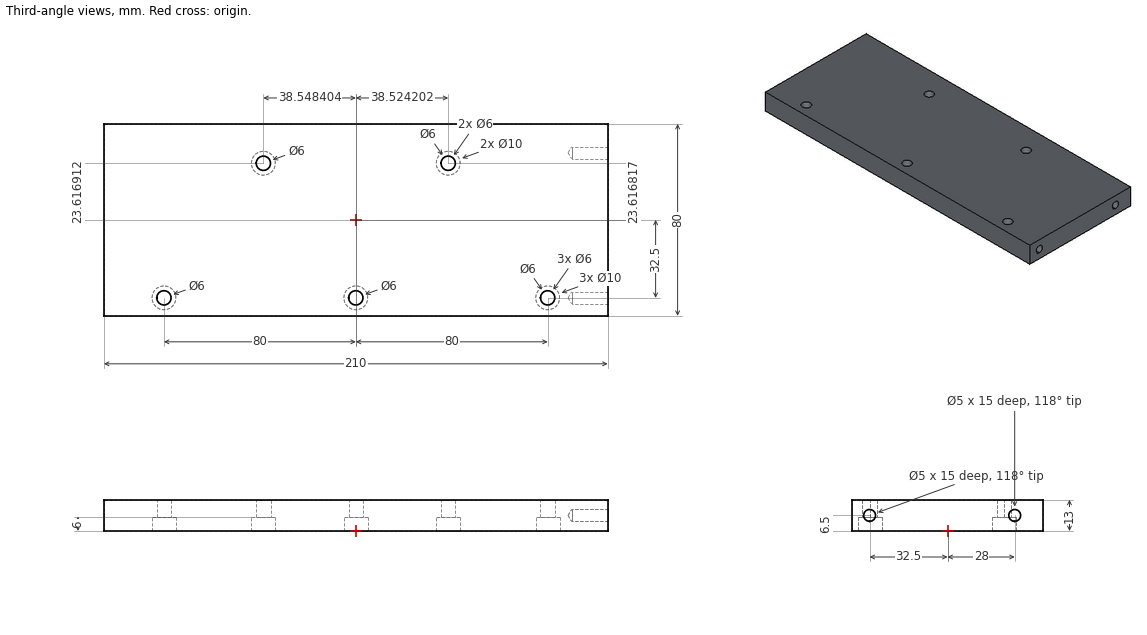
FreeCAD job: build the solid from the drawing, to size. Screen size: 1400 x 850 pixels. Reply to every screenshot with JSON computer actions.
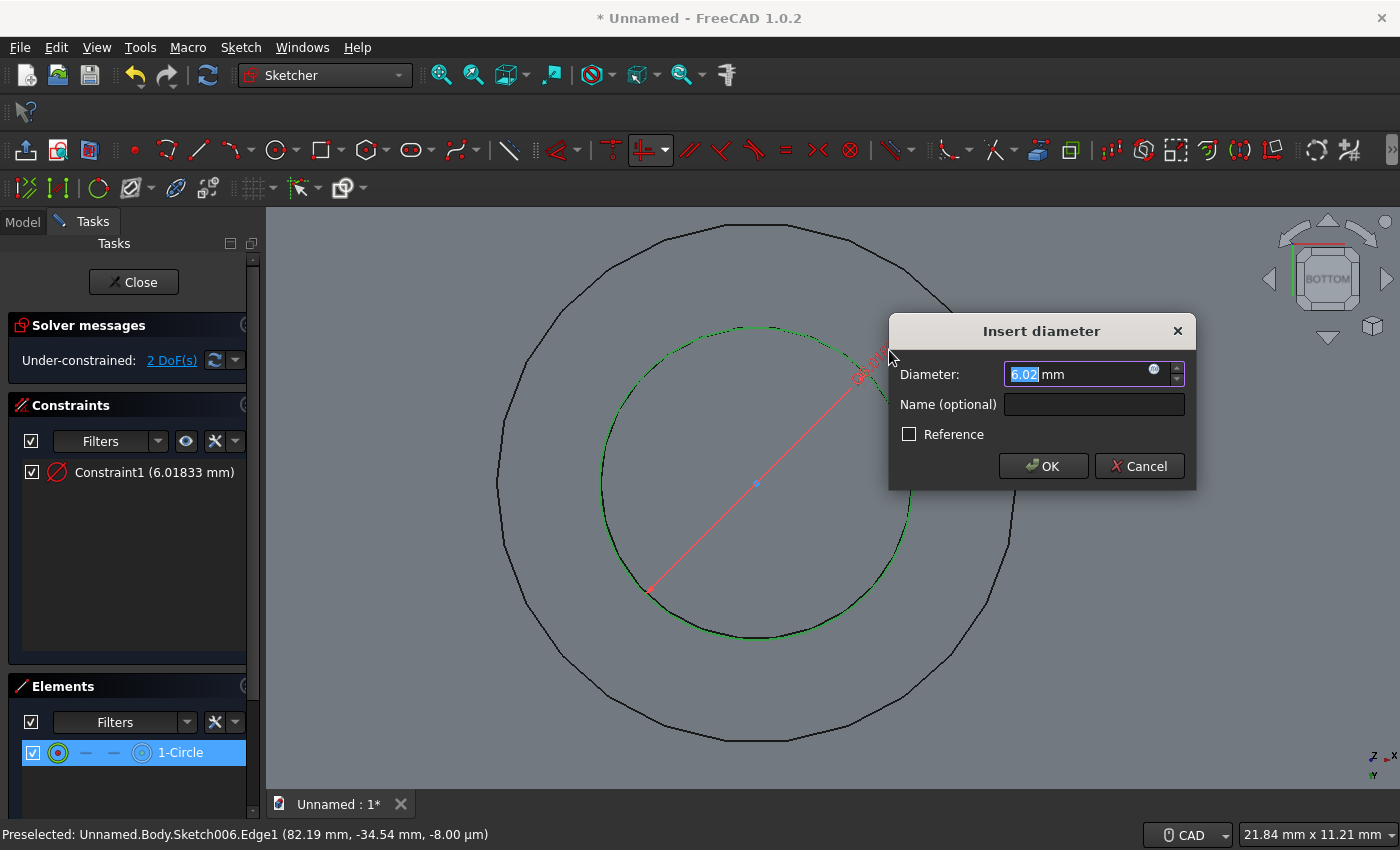
{"action": "type", "text": "6"}
{"action": "key", "text": "Return"}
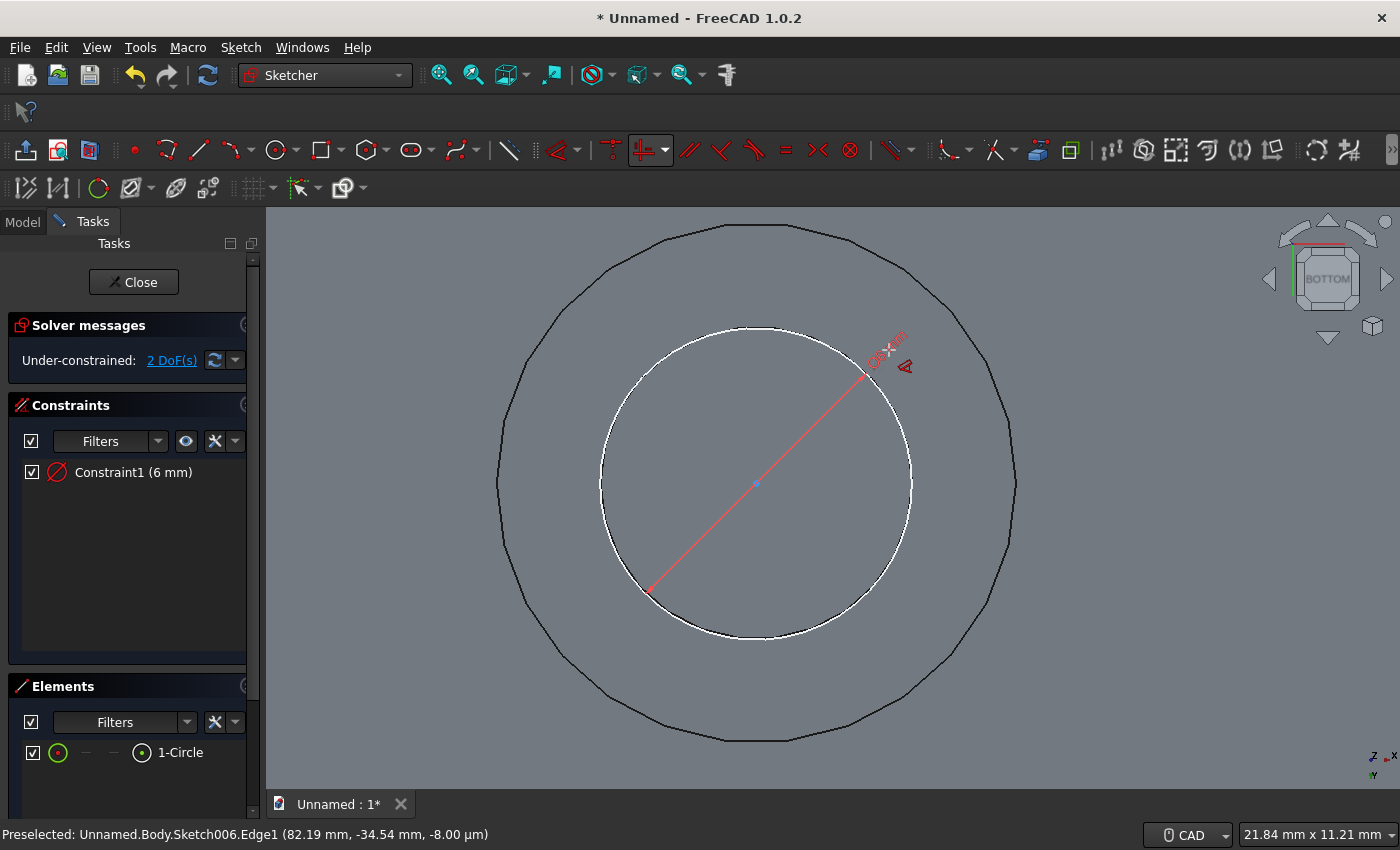
{"action": "left_click", "coordinate": [756, 484]}
{"action": "left_click", "coordinate": [525, 450]}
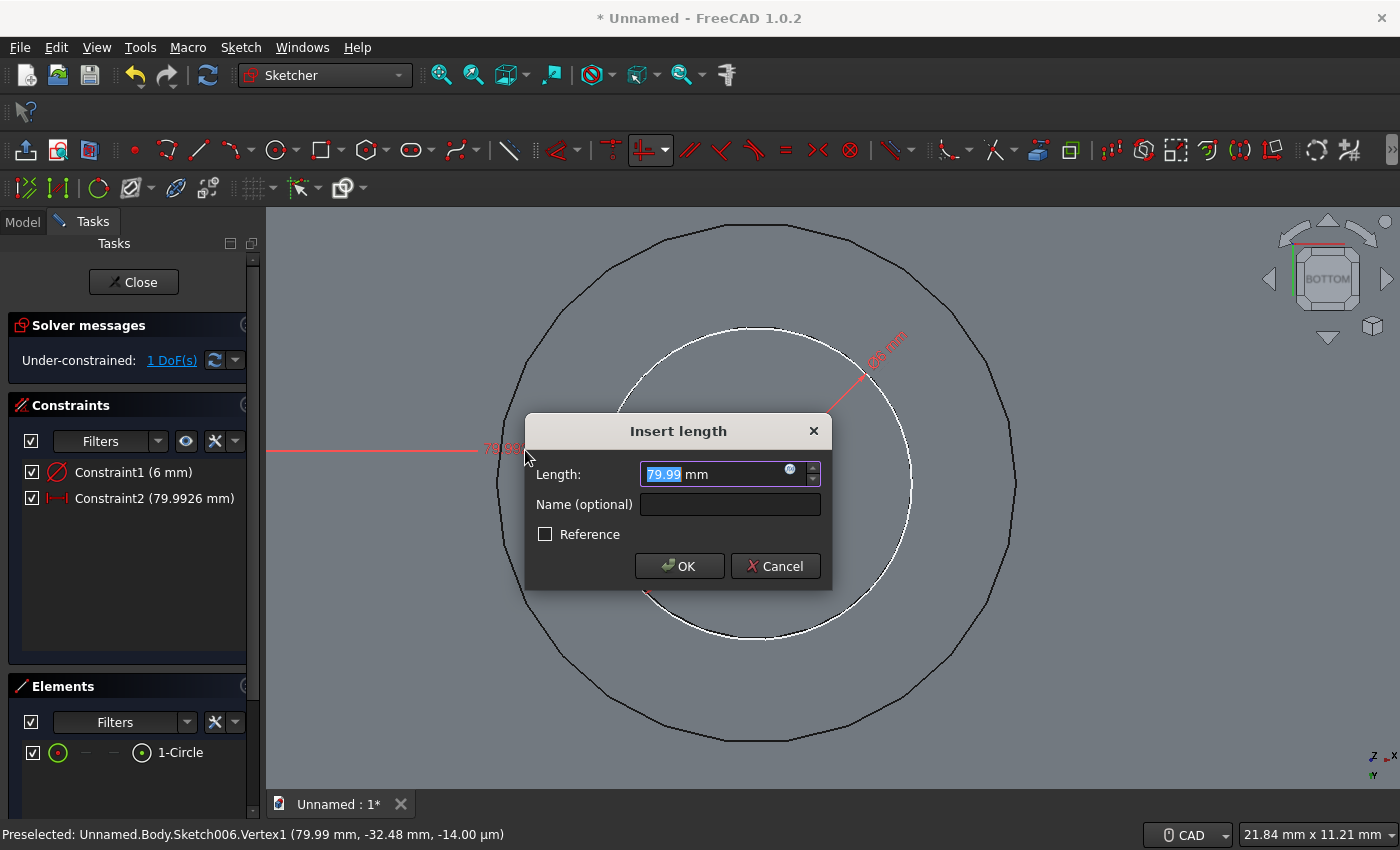
{"action": "type", "text": "80"}
{"action": "key", "text": "Return"}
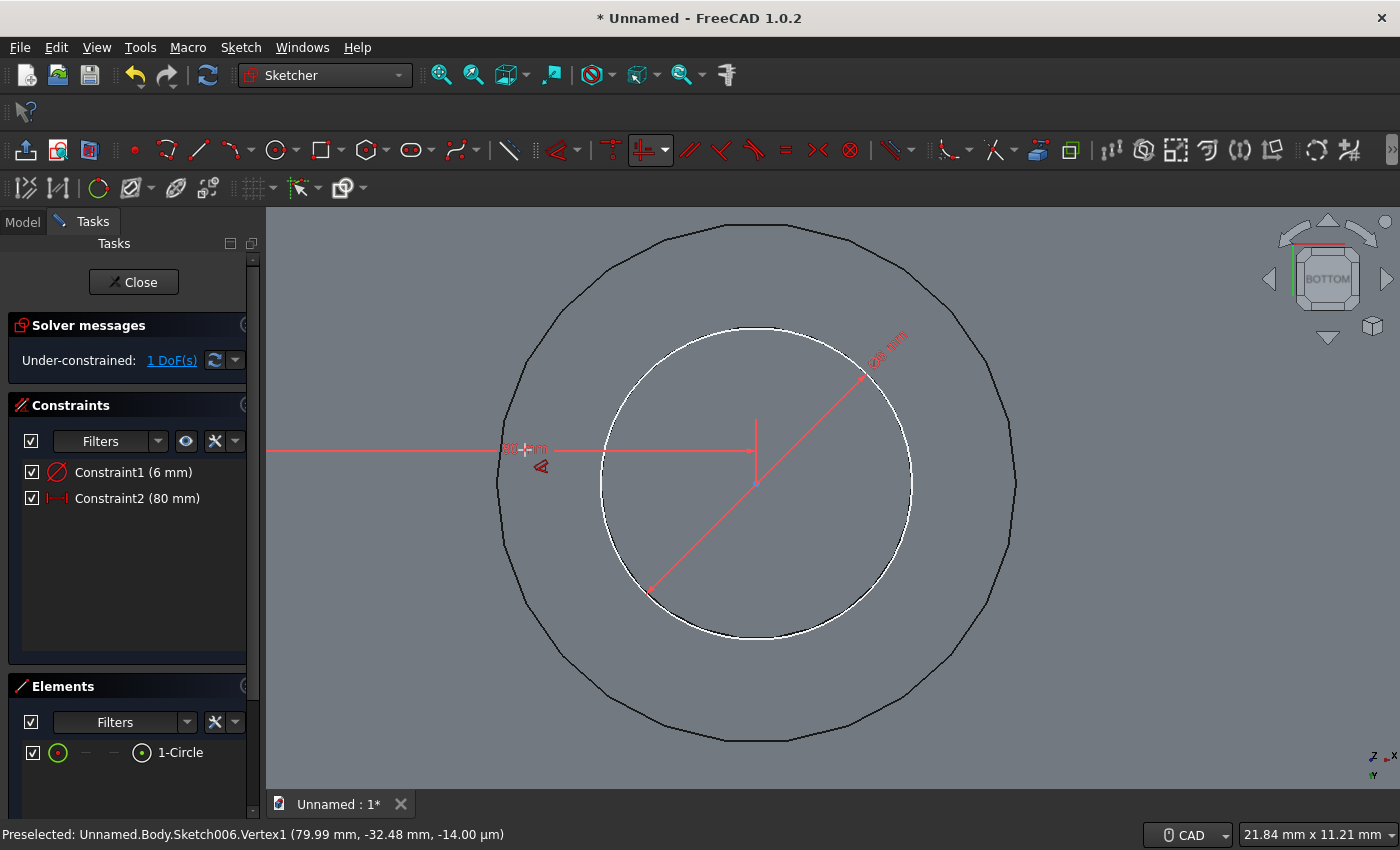
{"action": "left_click", "coordinate": [756, 484]}
{"action": "left_click", "coordinate": [790, 622]}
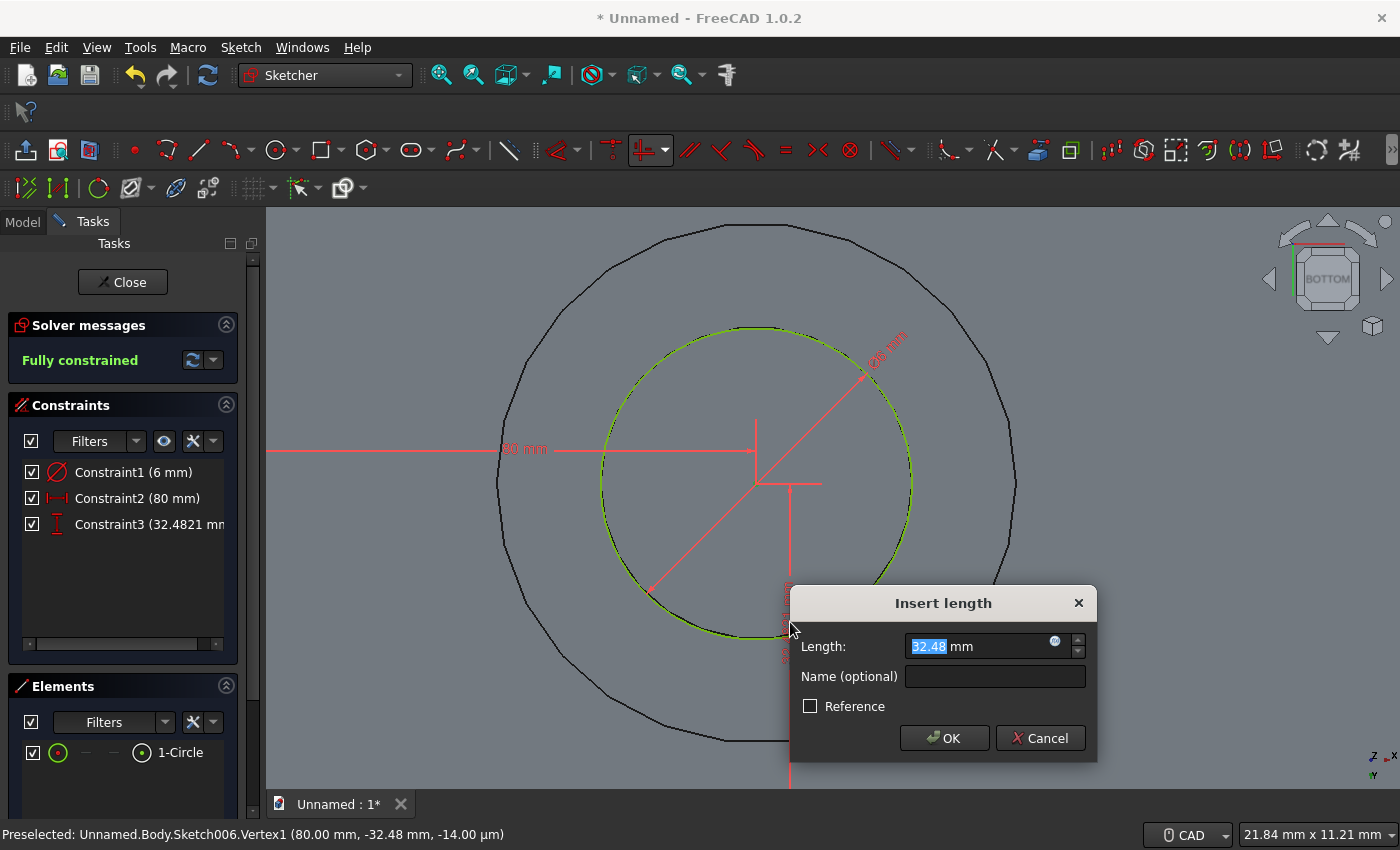
{"action": "type", "text": "32.5"}
{"action": "key", "text": "Return"}
{"action": "key", "text": "Escape"}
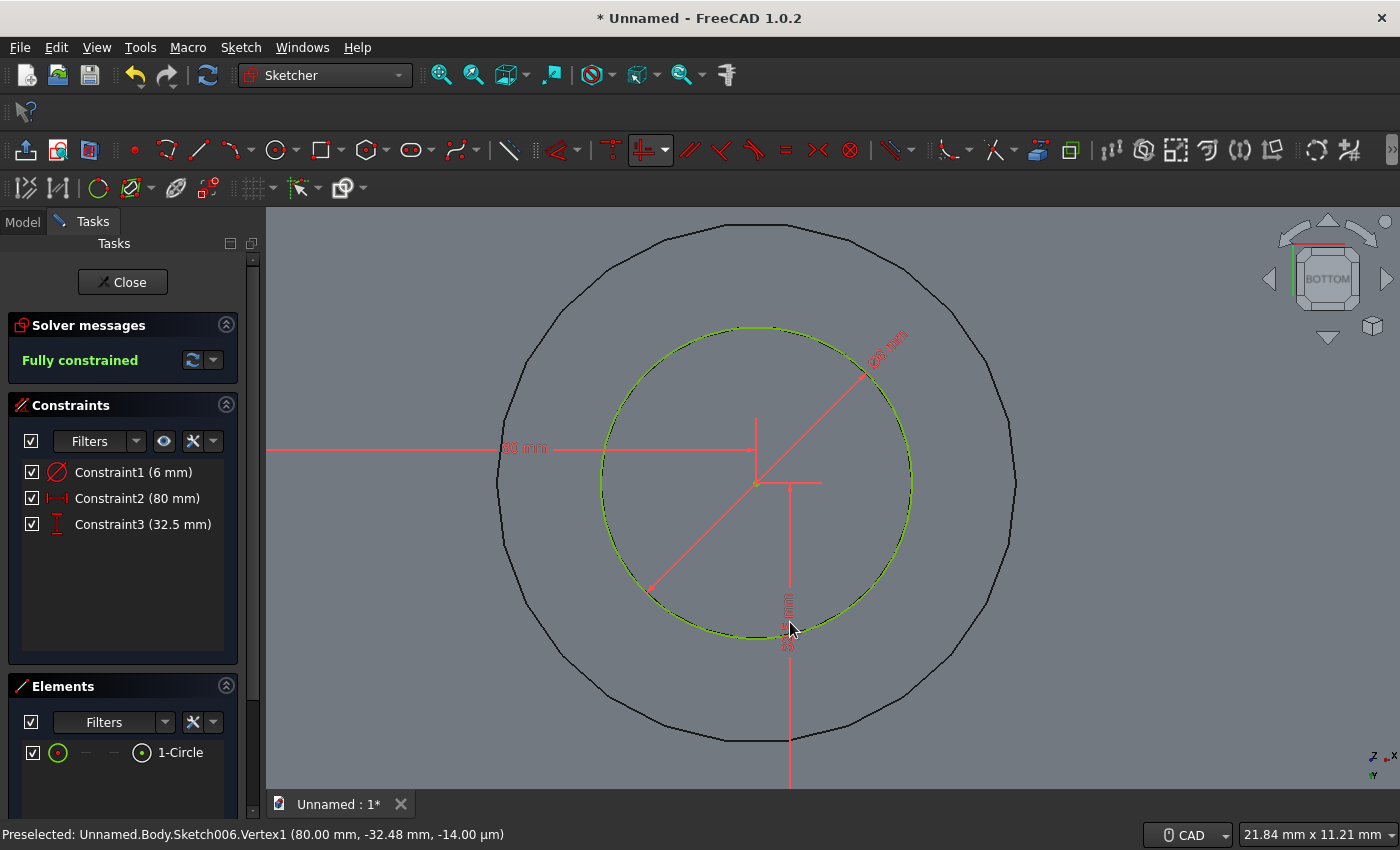
{"action": "left_click", "coordinate": [123, 282]}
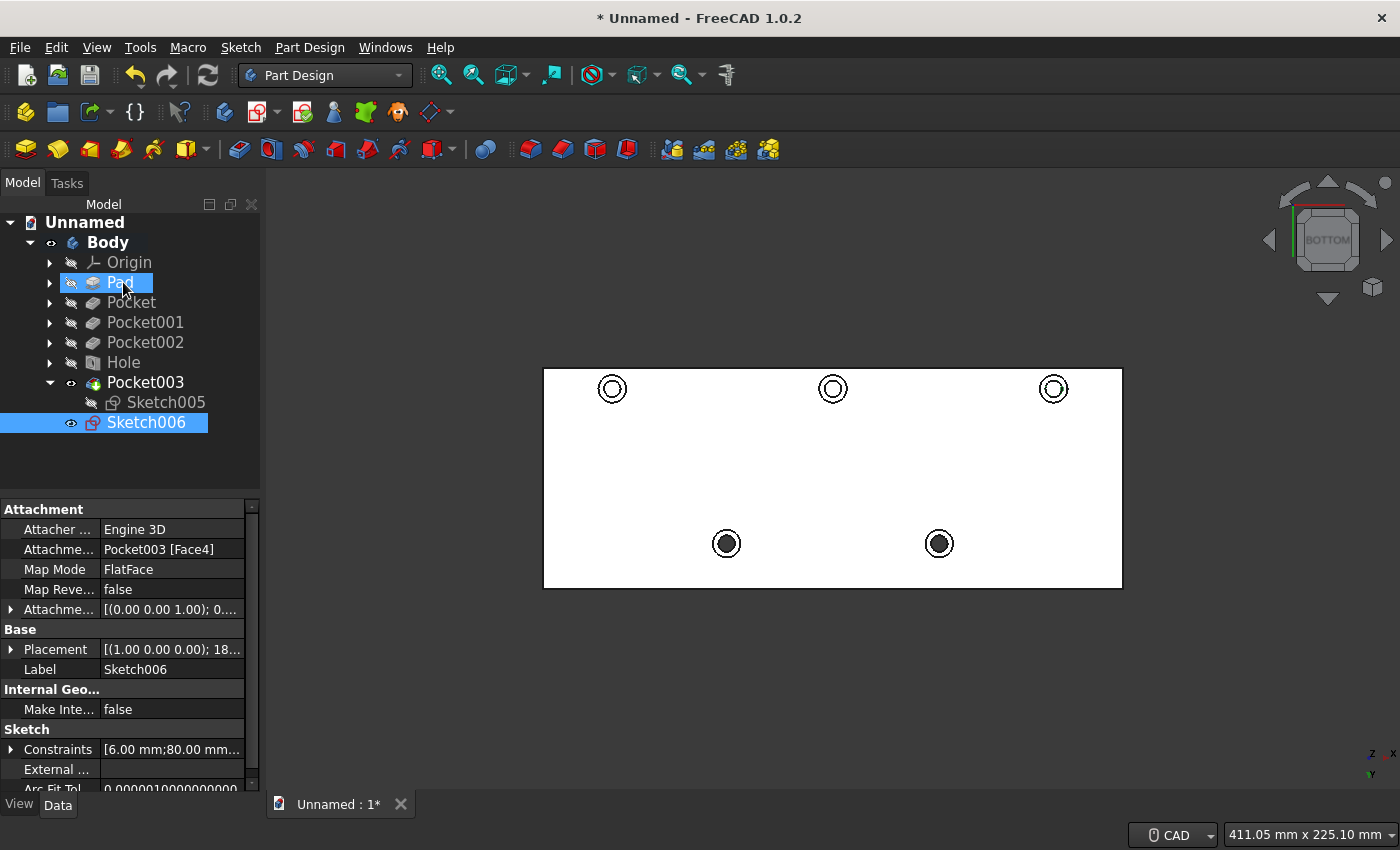
{"action": "left_click", "coordinate": [240, 150]}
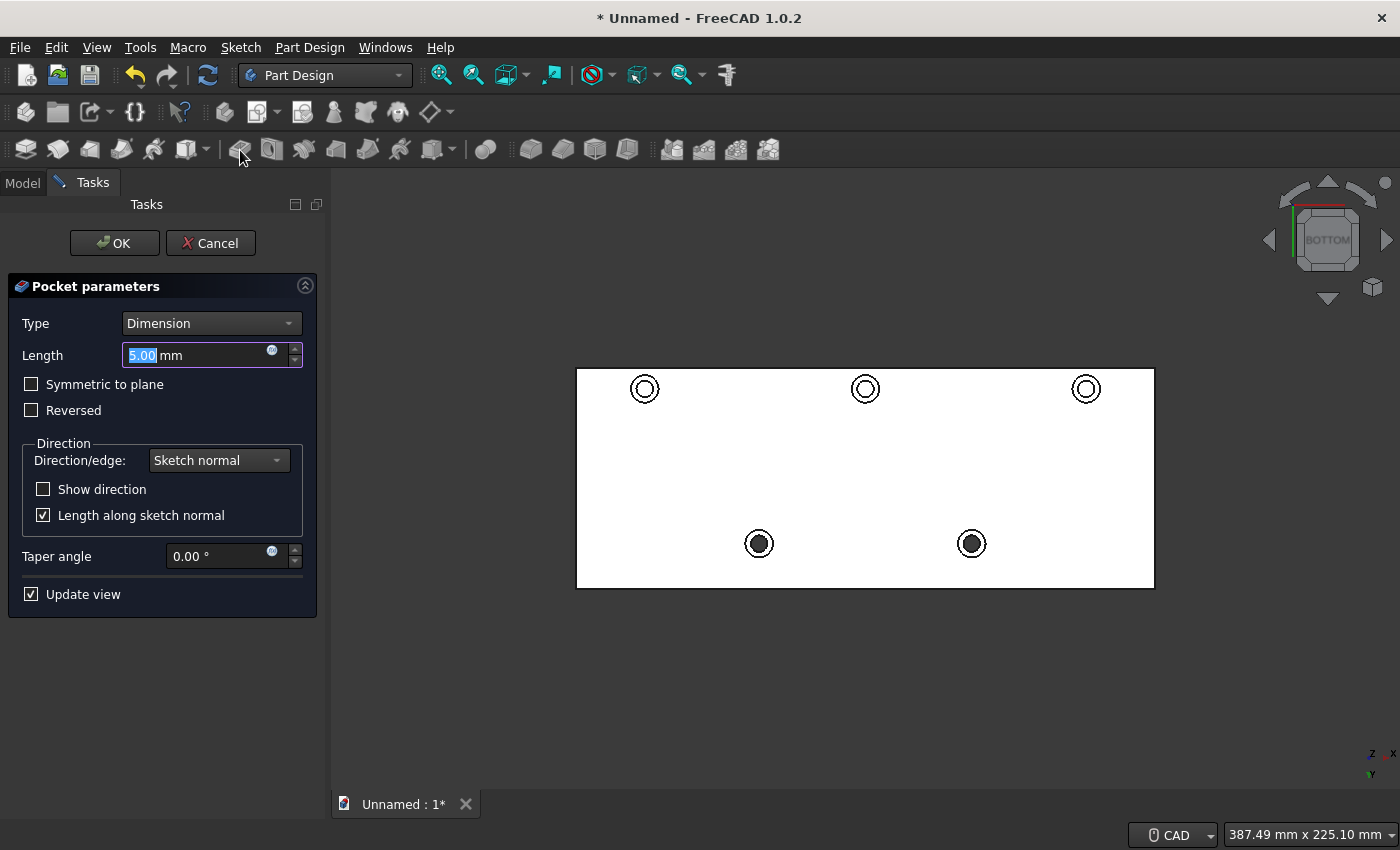
{"action": "left_click", "coordinate": [212, 324]}